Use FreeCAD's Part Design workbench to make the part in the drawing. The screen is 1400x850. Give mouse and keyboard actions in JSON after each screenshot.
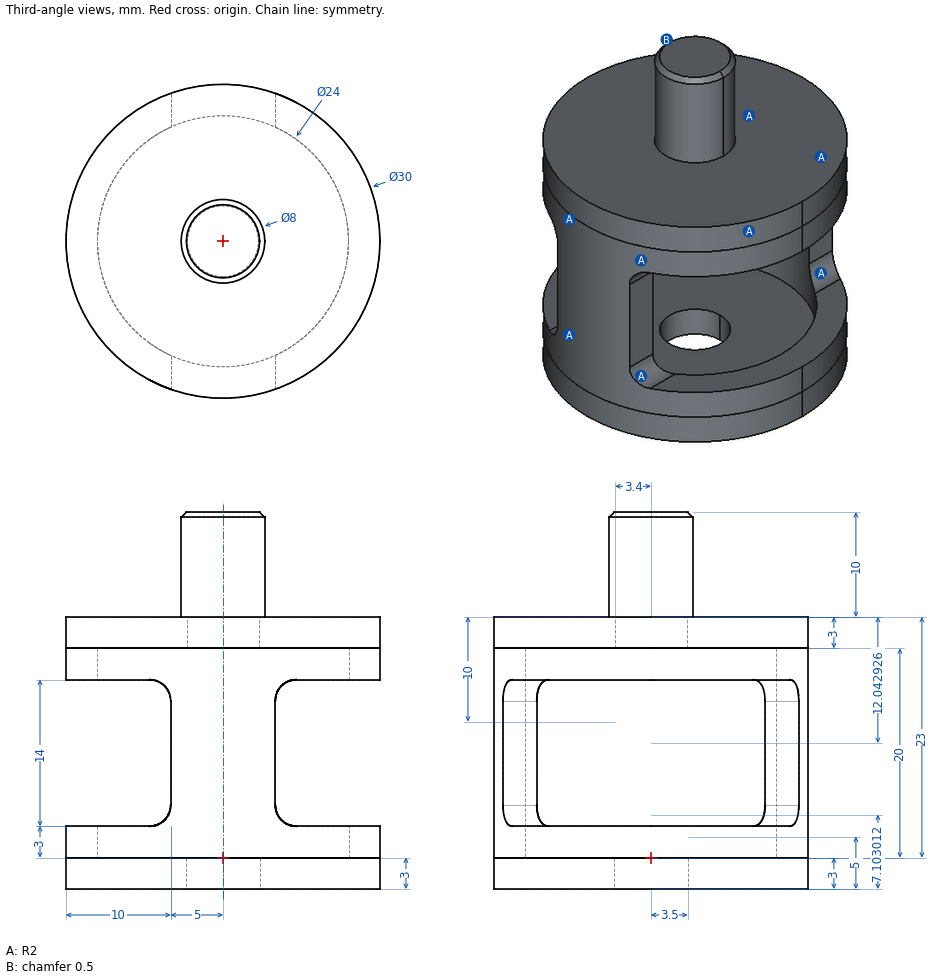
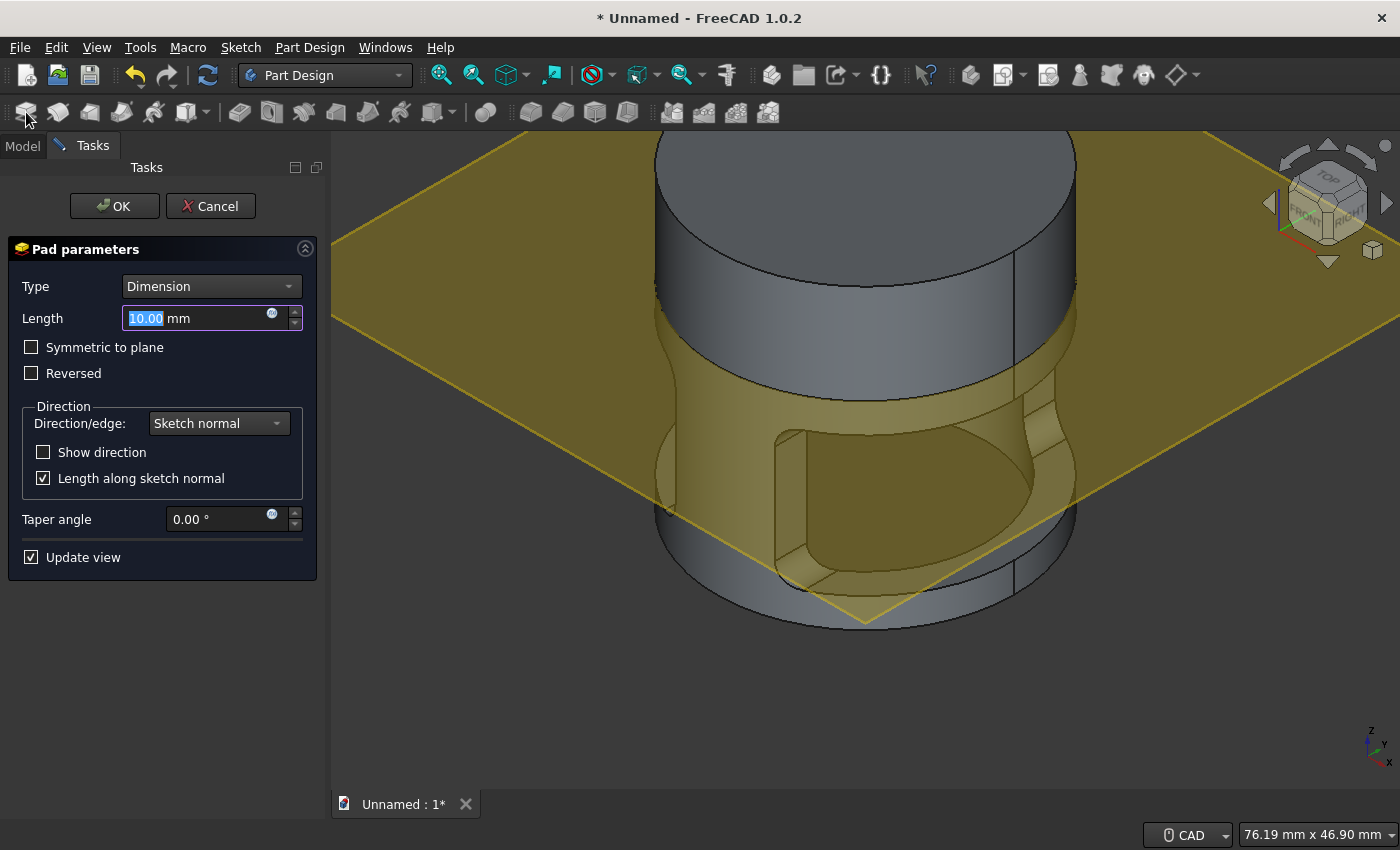
{"action": "type", "text": "3"}
{"action": "key", "text": "Tab"}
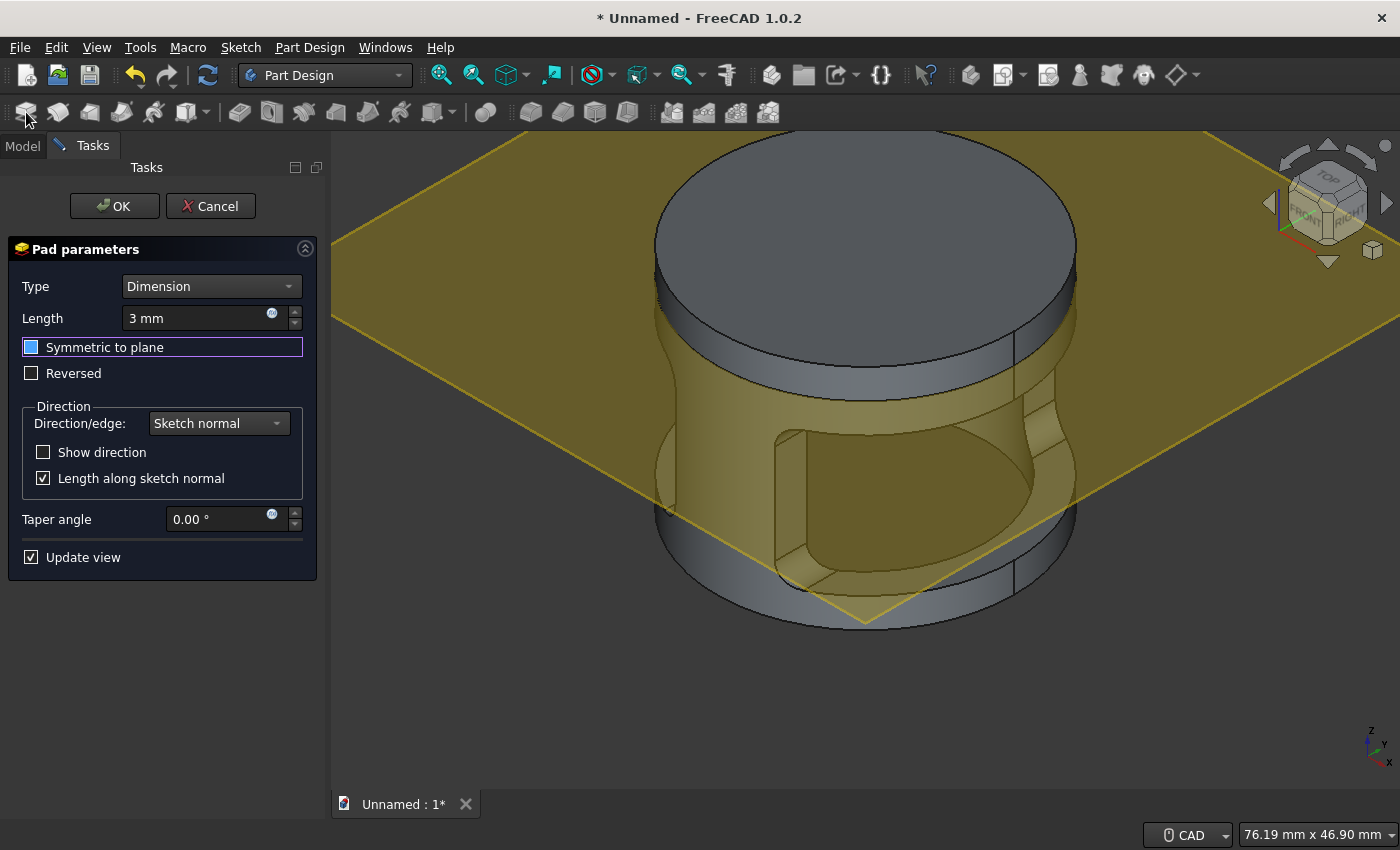
{"action": "left_click", "coordinate": [115, 206]}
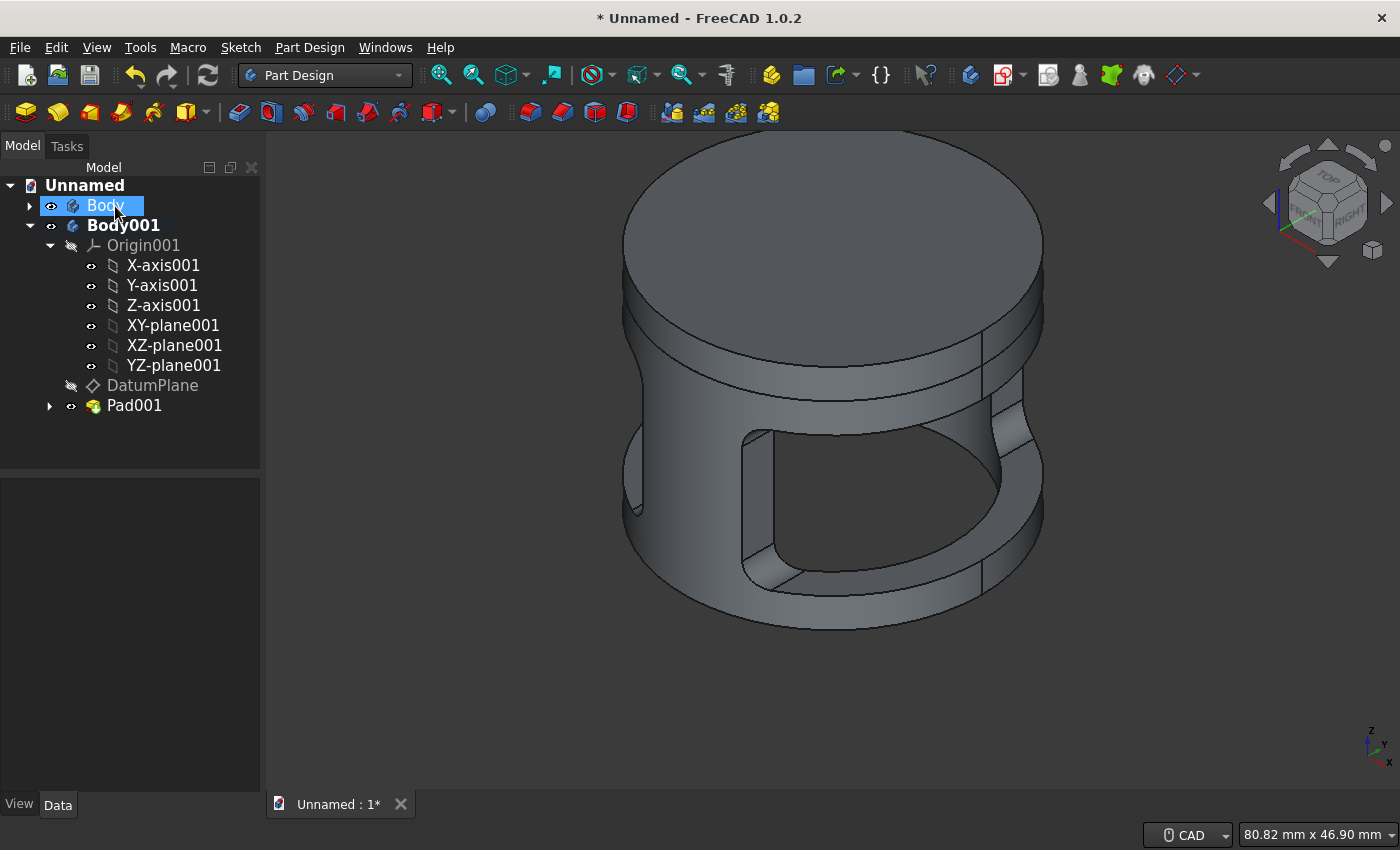
{"action": "key", "text": "v f"}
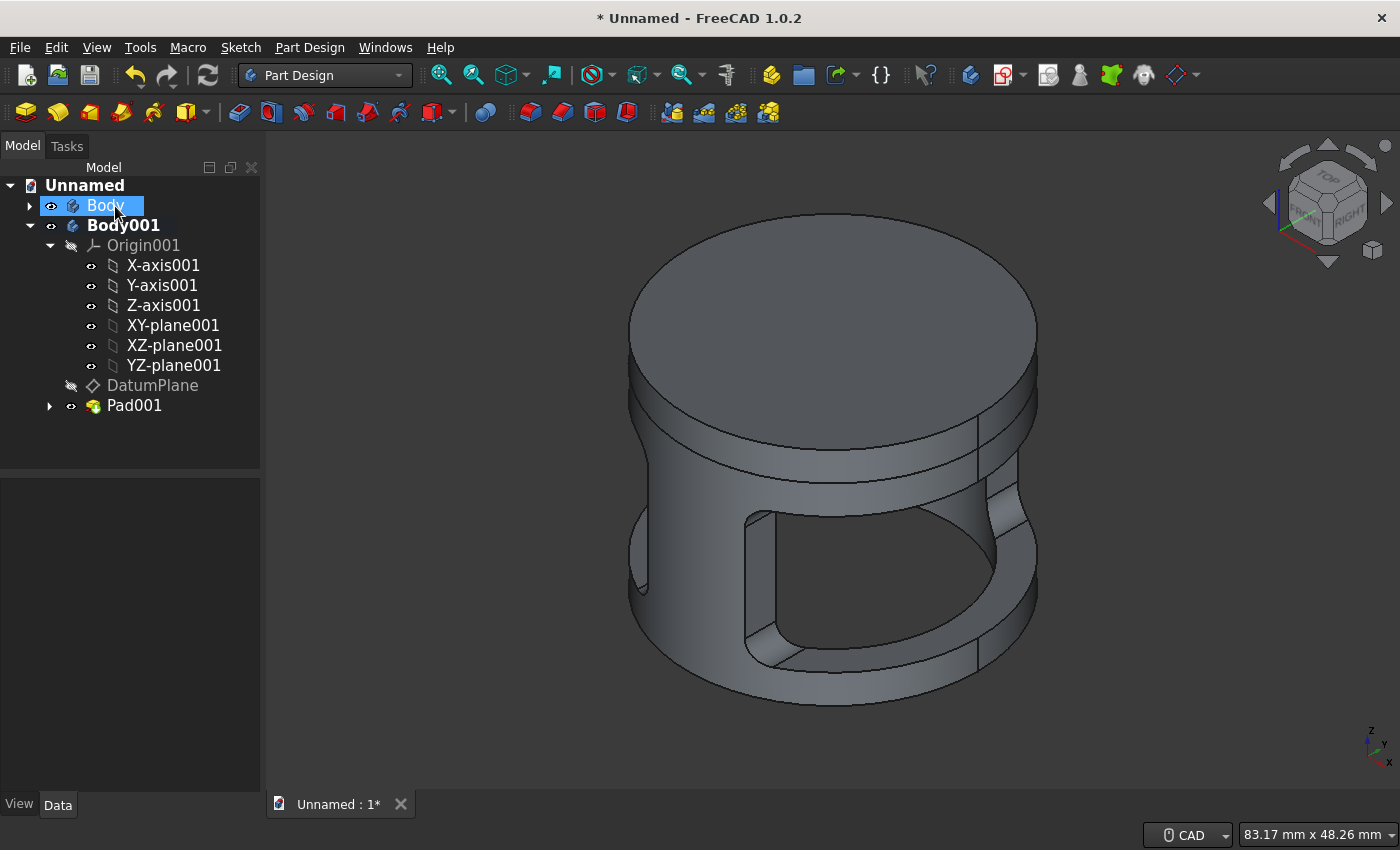
{"action": "left_click", "coordinate": [1004, 76]}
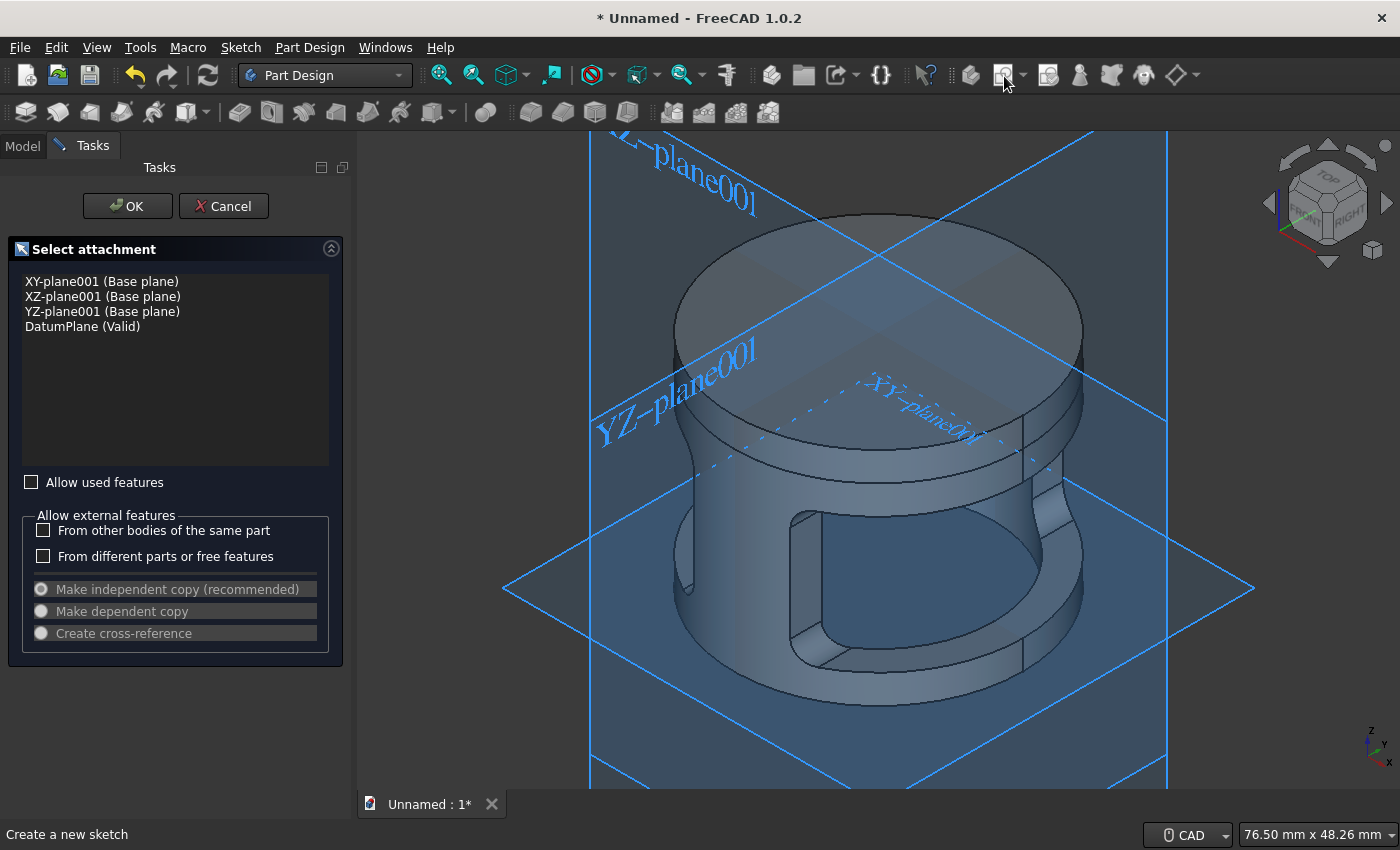
{"action": "left_click", "coordinate": [82, 312]}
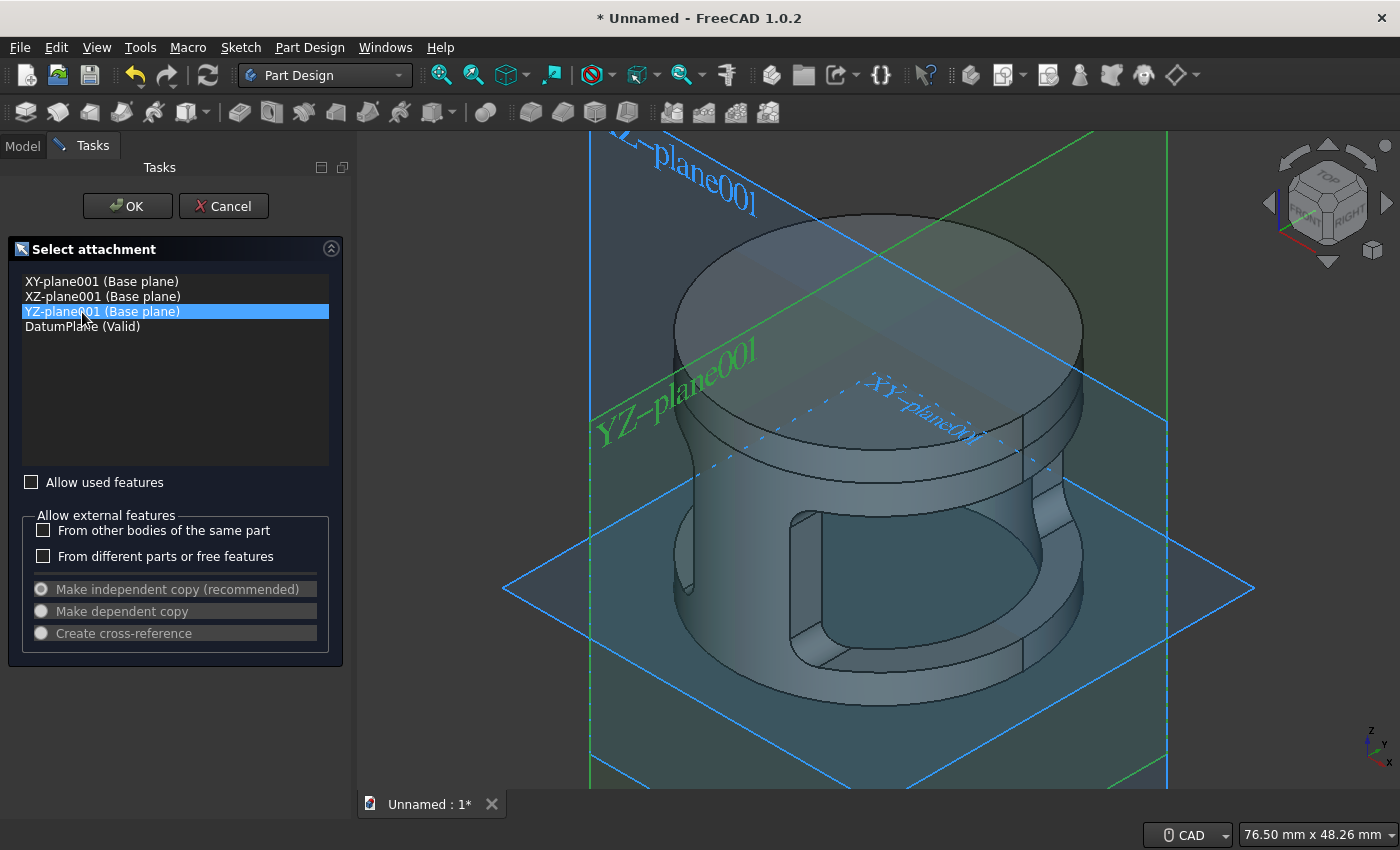
{"action": "left_click", "coordinate": [128, 206]}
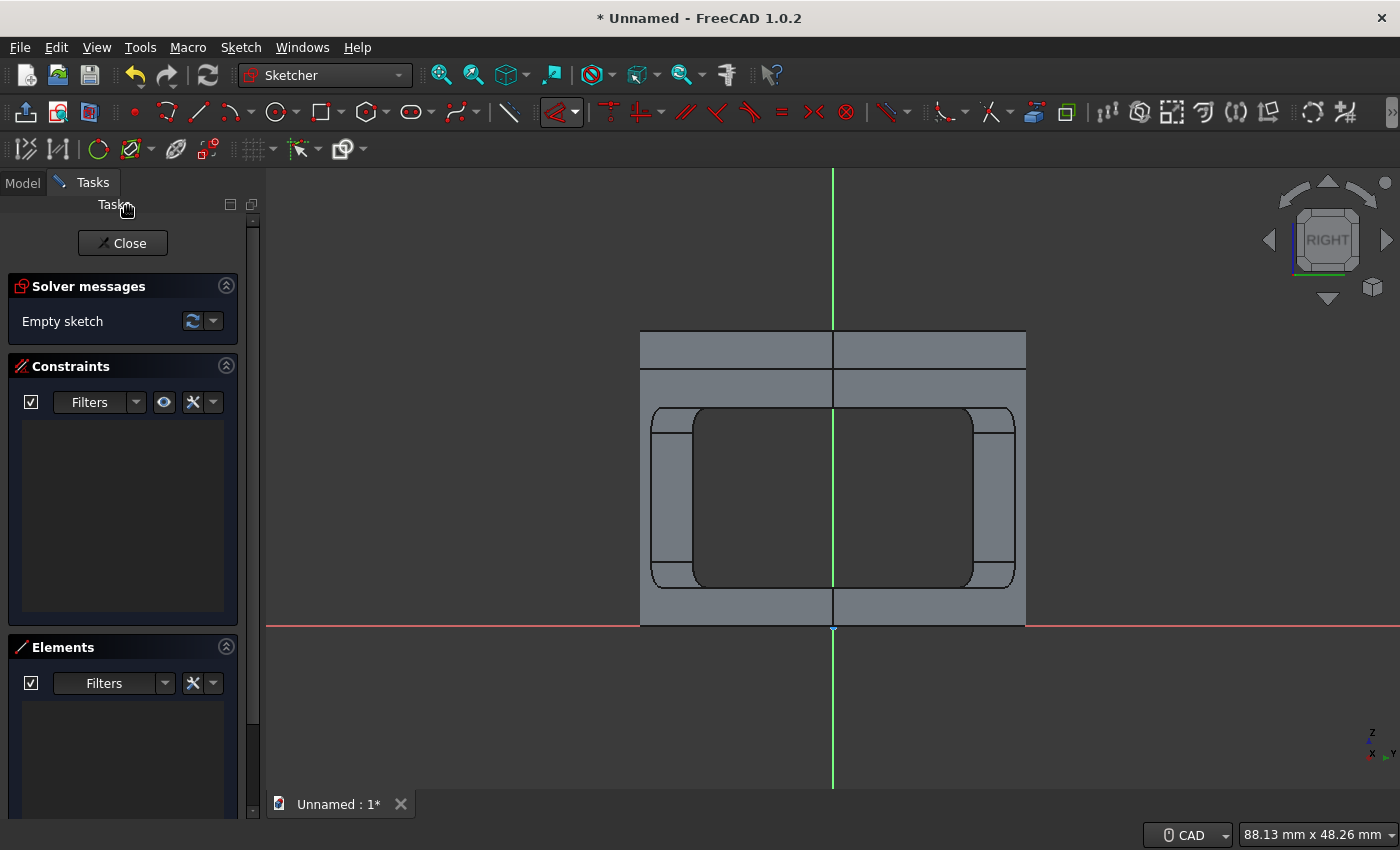
{"action": "key", "text": "q s"}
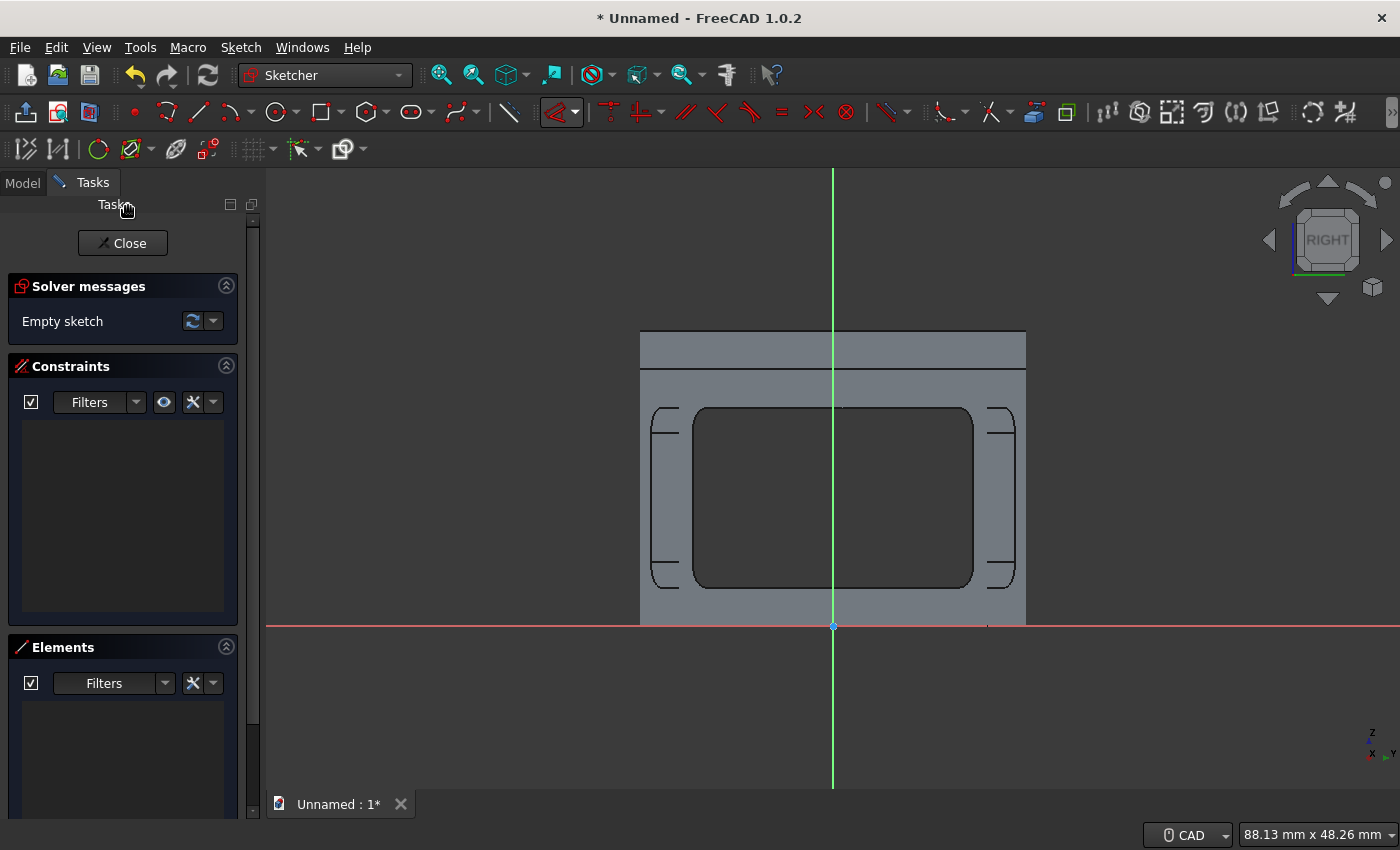
{"action": "key", "text": "g m"}